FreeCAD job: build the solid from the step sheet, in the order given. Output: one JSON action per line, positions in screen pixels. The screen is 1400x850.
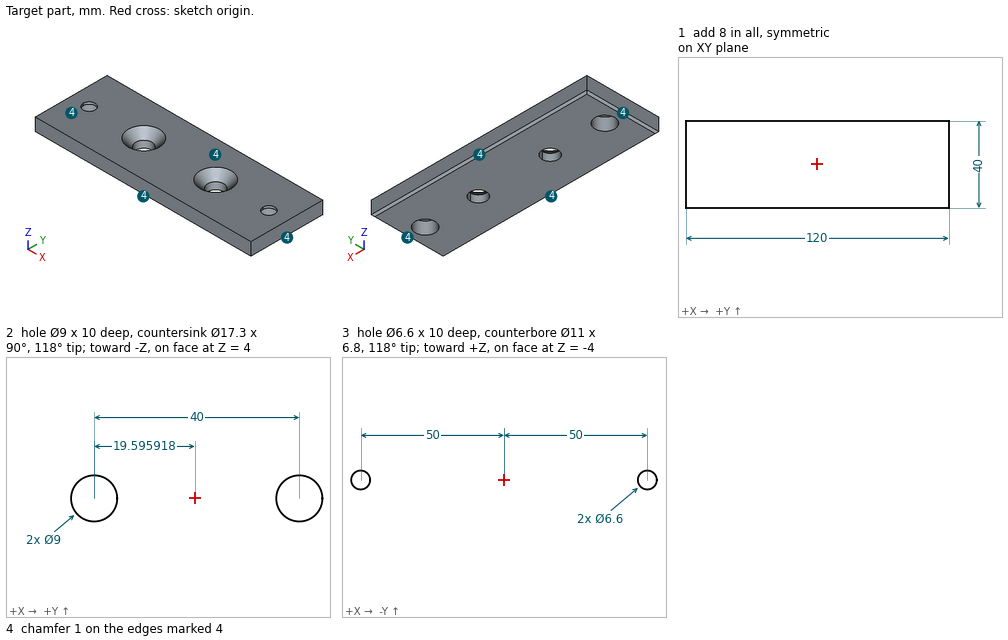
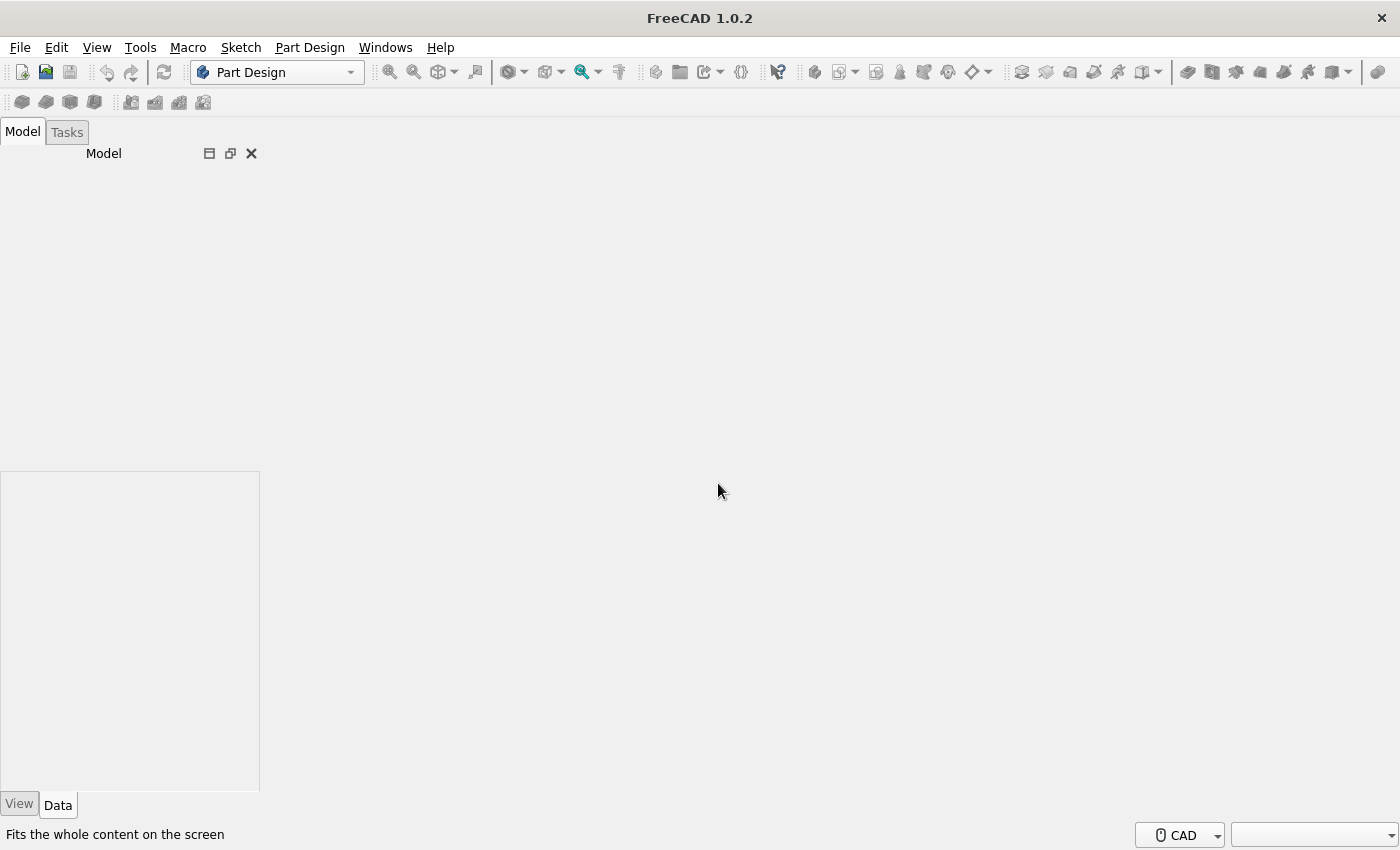
{"action": "left_click", "coordinate": [22, 72]}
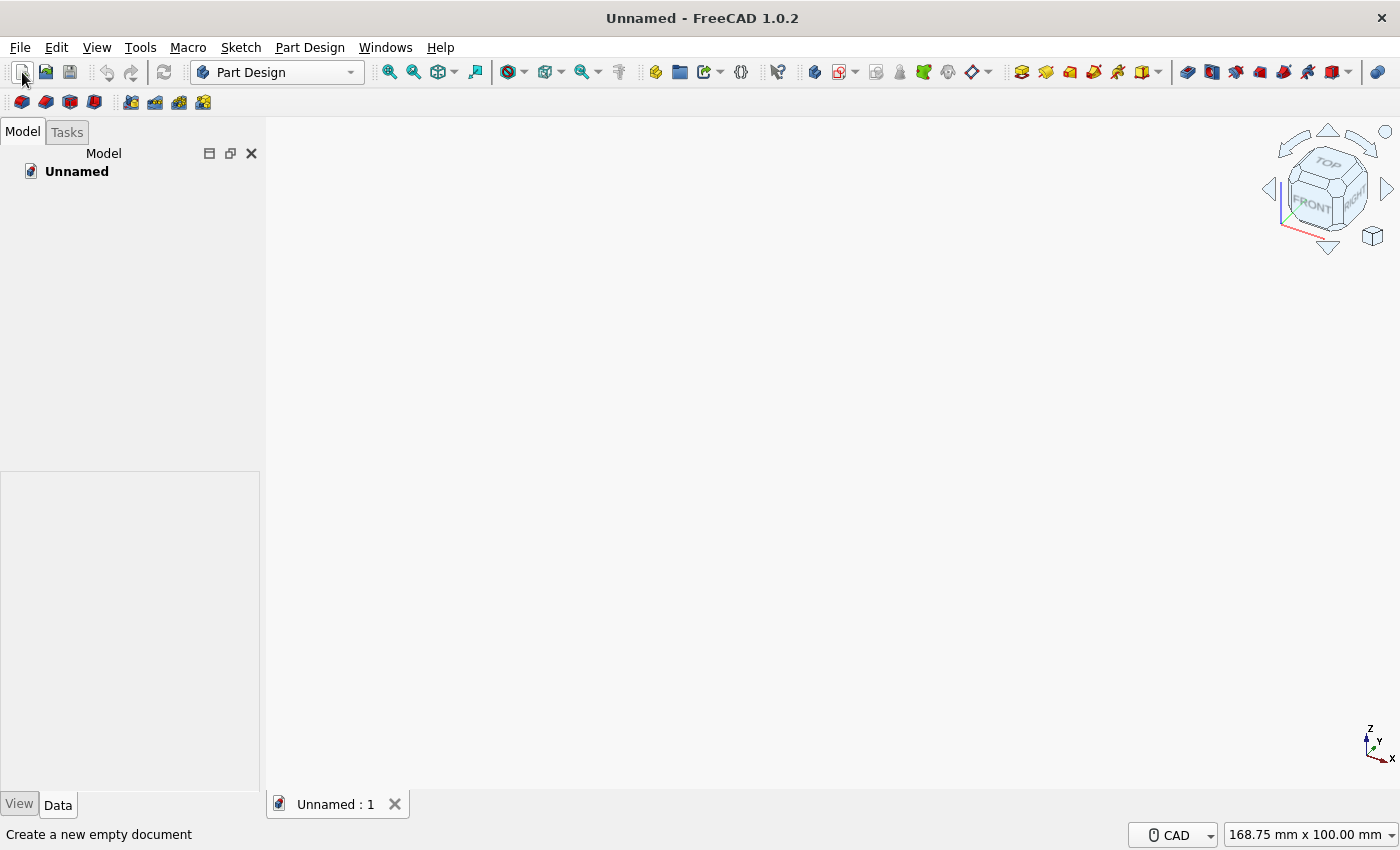
{"action": "left_click", "coordinate": [840, 72]}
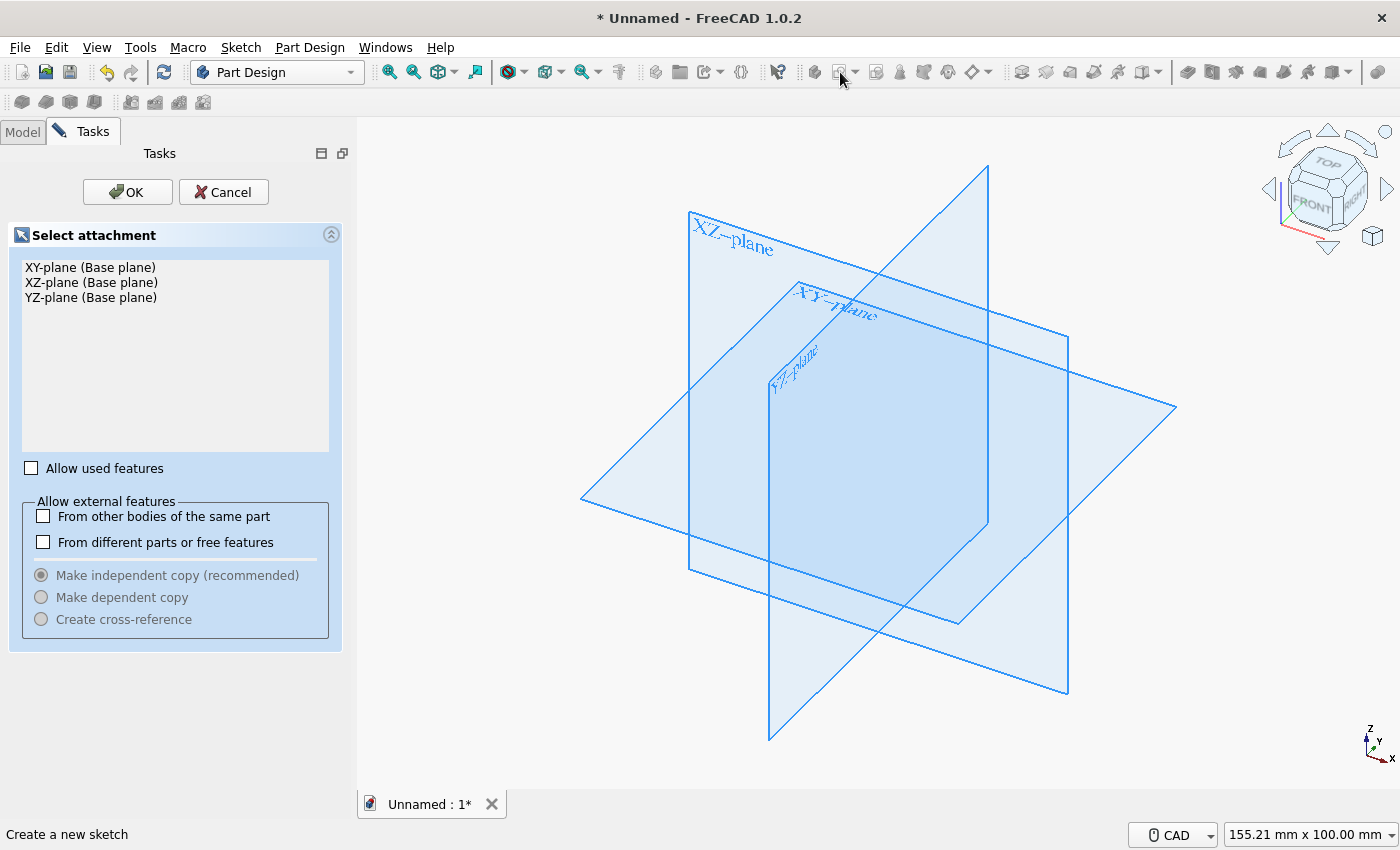
{"action": "left_click", "coordinate": [82, 268]}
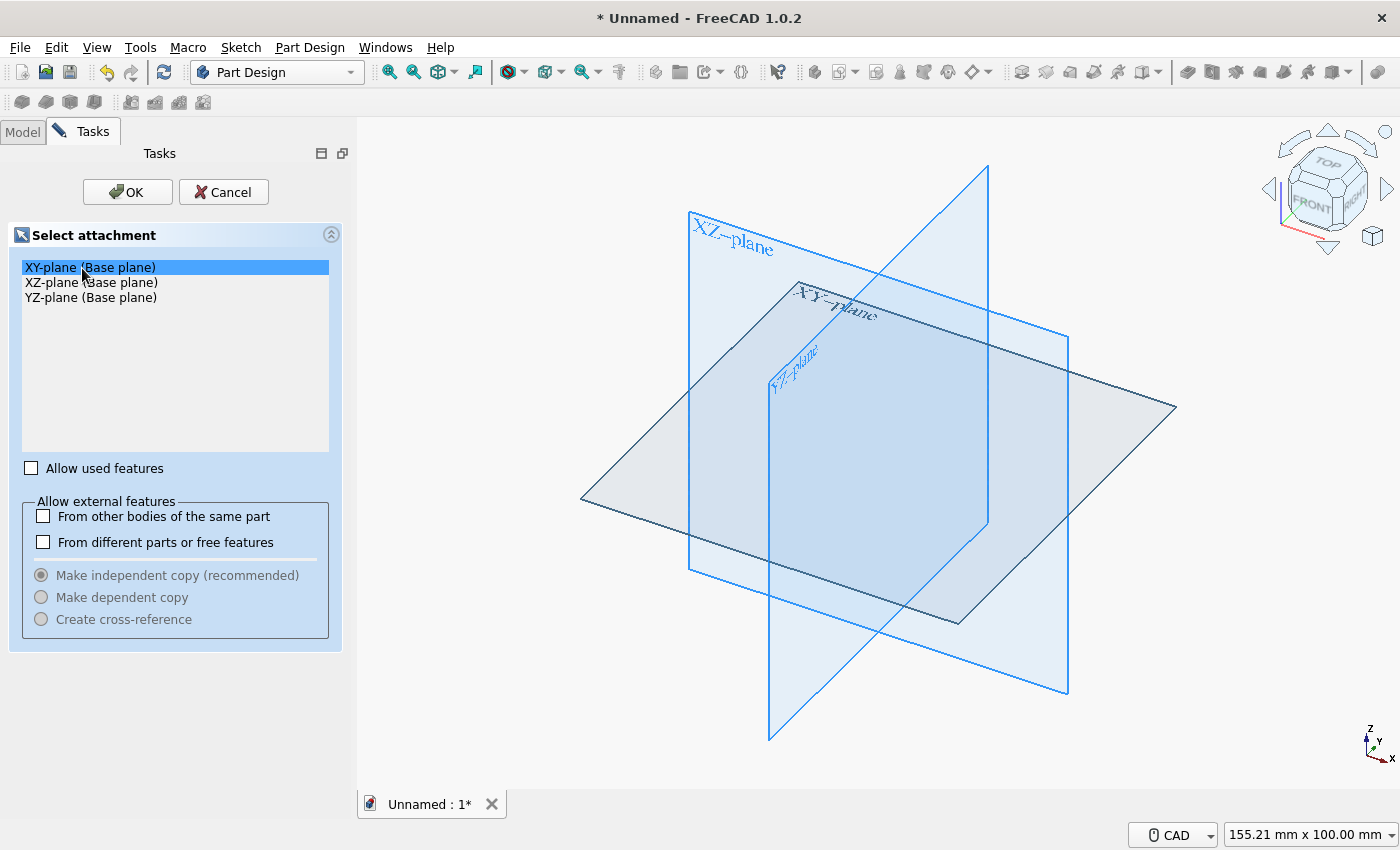
{"action": "left_click", "coordinate": [128, 192]}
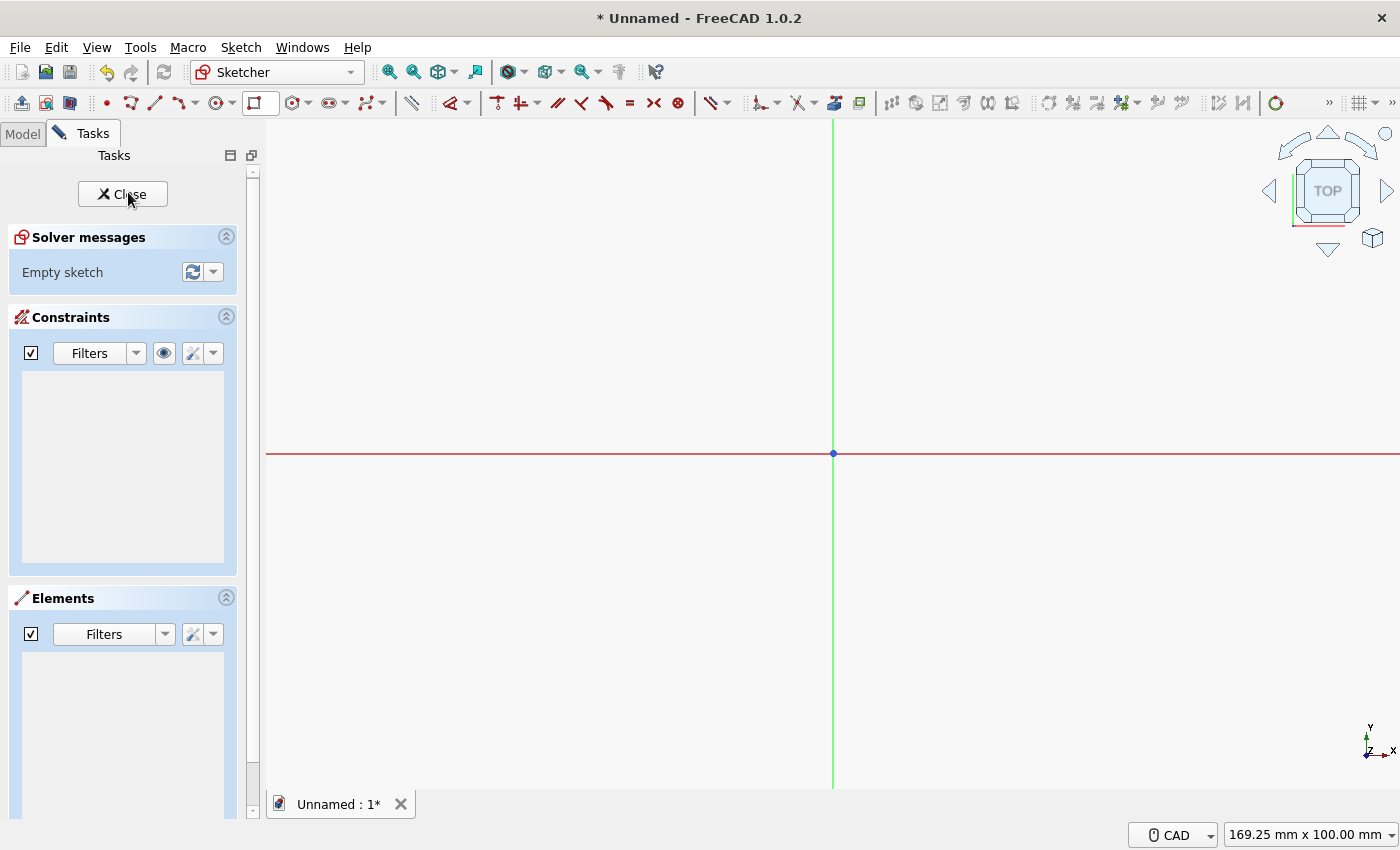
{"action": "scroll", "coordinate": [455, 454], "scroll_direction": "down", "scroll_amount": 1}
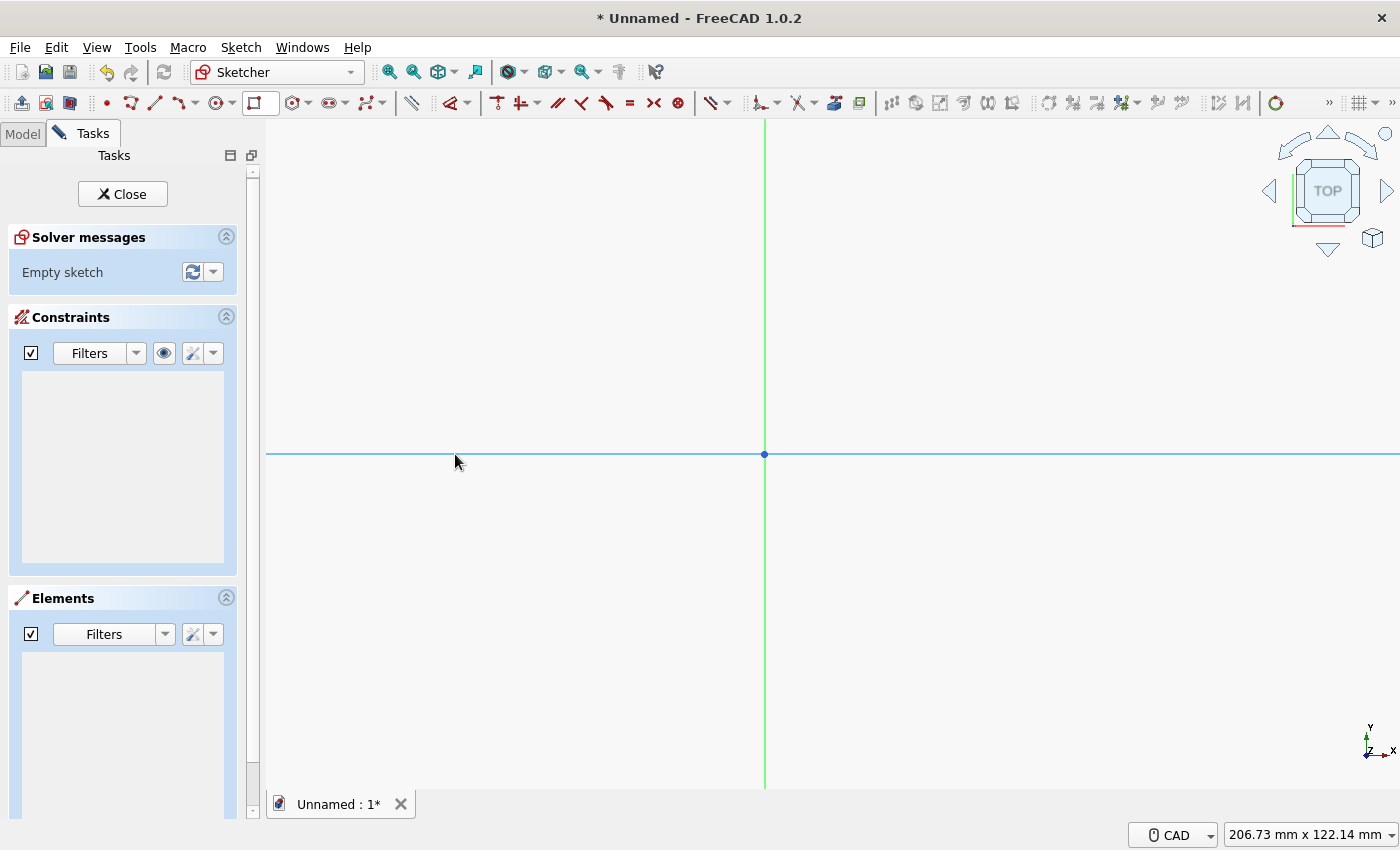
{"action": "left_click", "coordinate": [274, 104]}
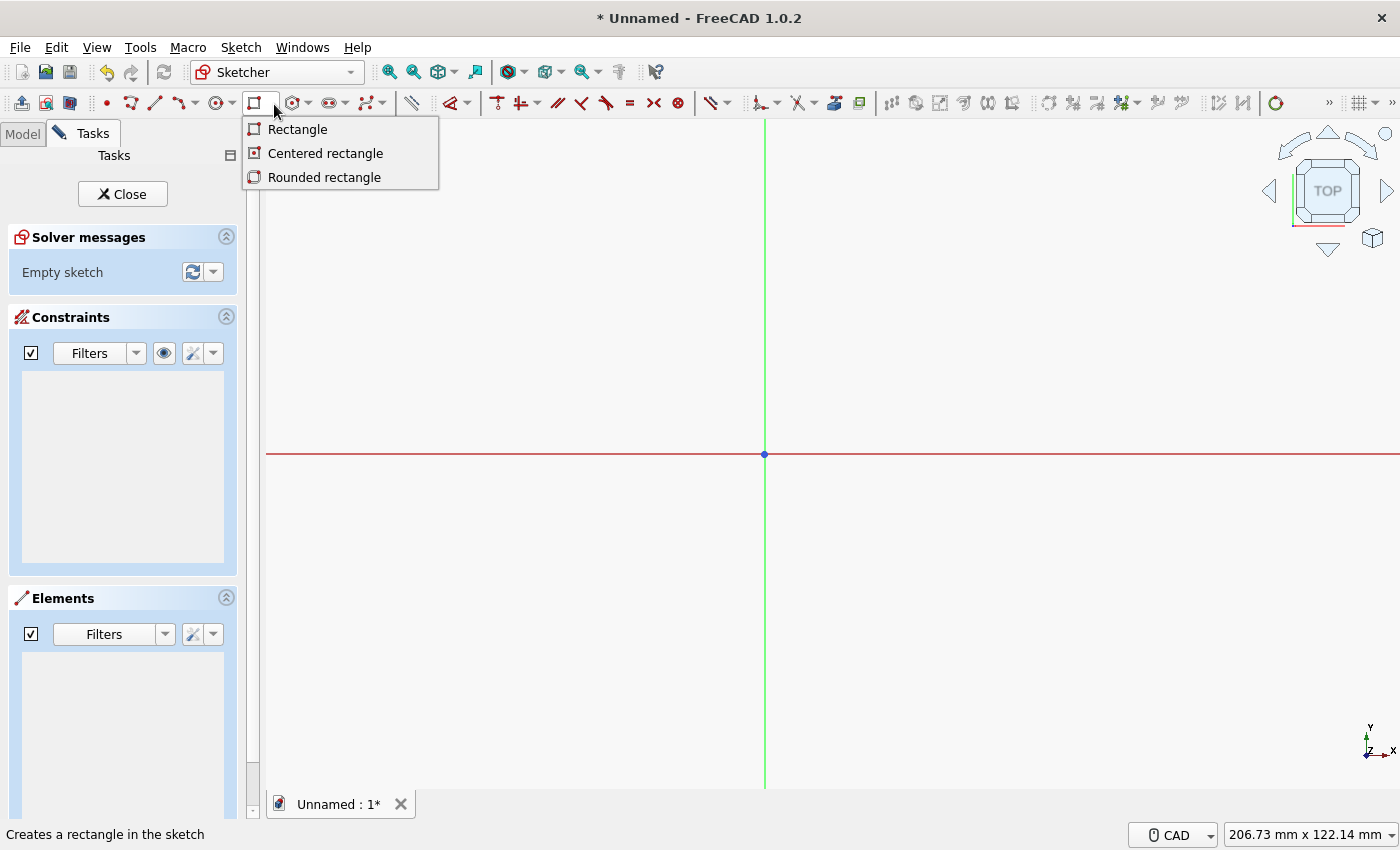
{"action": "left_click", "coordinate": [340, 153]}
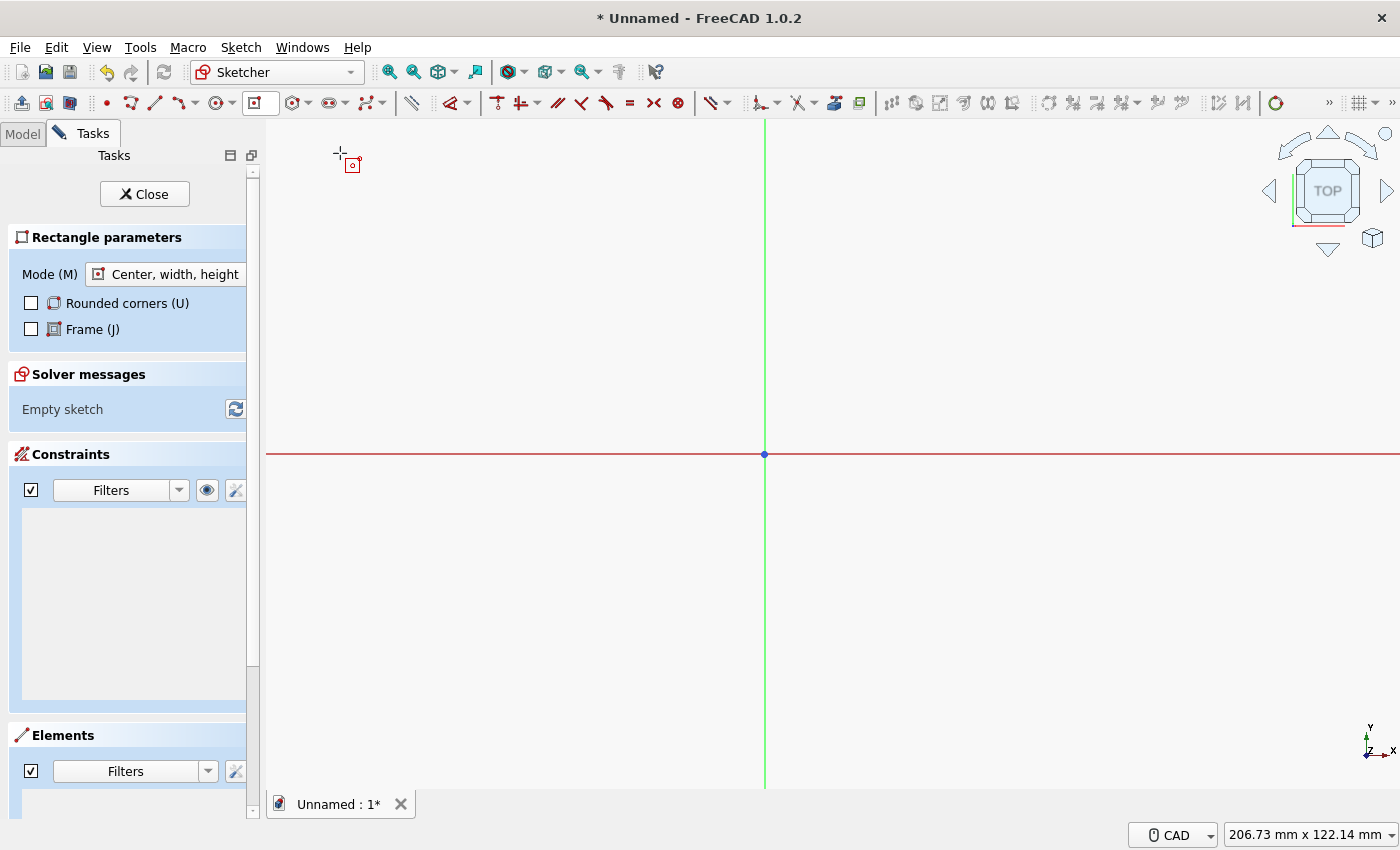
{"action": "left_click", "coordinate": [765, 454]}
{"action": "left_click", "coordinate": [1094, 344]}
{"action": "key", "text": "Escape"}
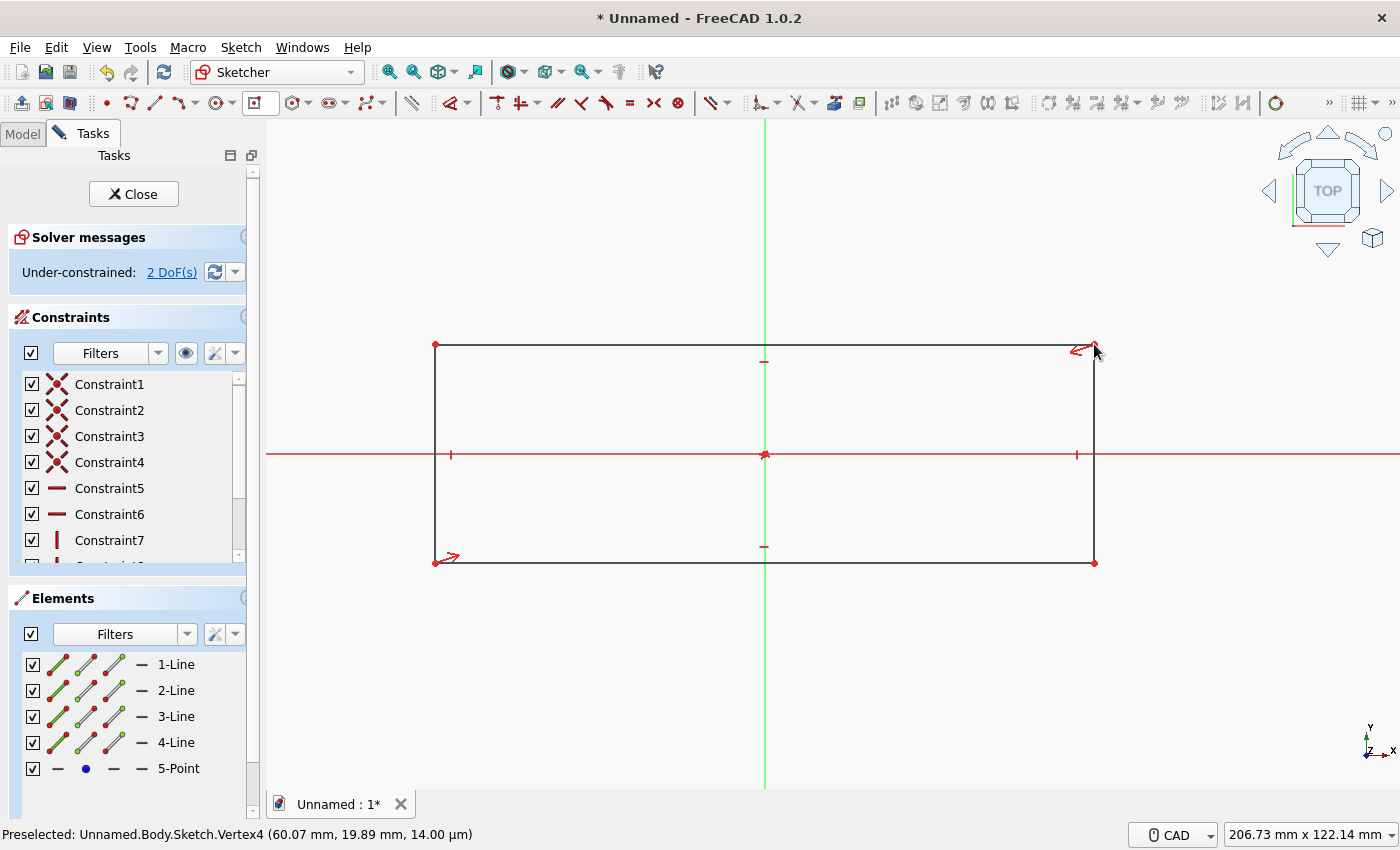
{"action": "left_click", "coordinate": [1094, 498]}